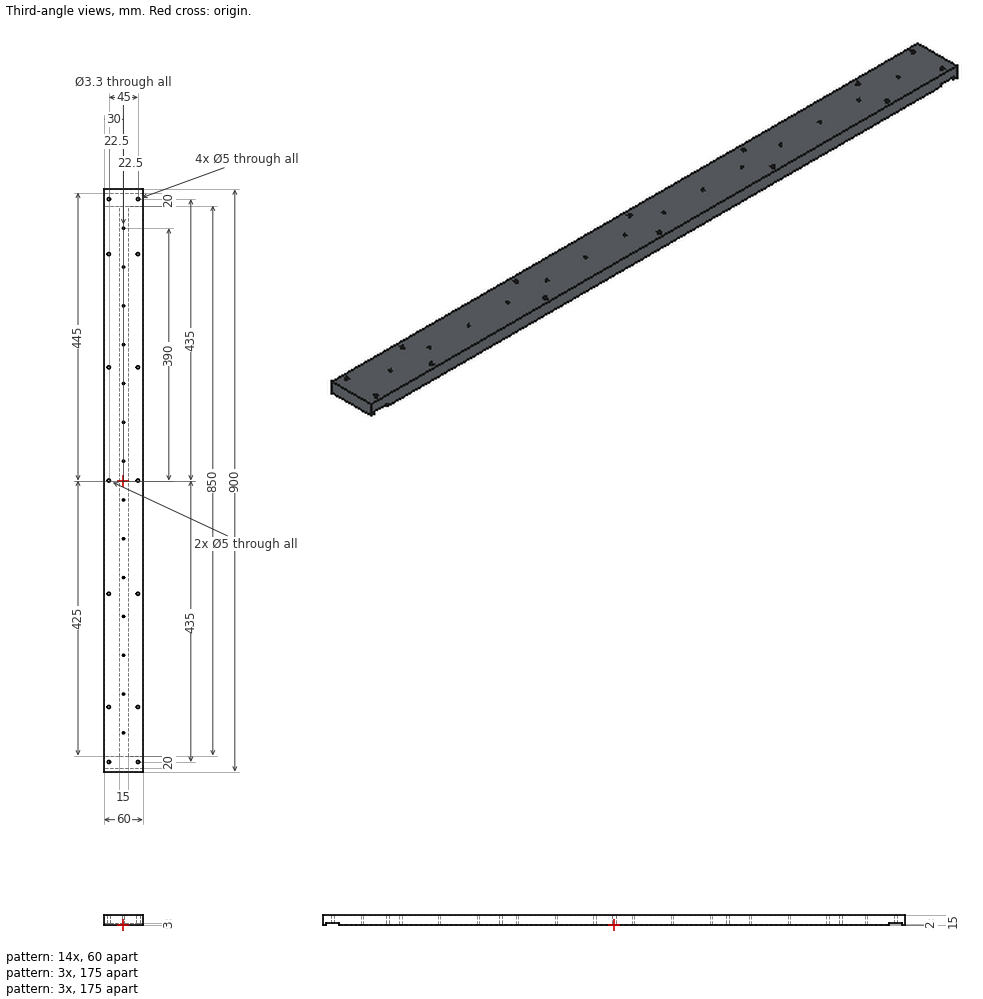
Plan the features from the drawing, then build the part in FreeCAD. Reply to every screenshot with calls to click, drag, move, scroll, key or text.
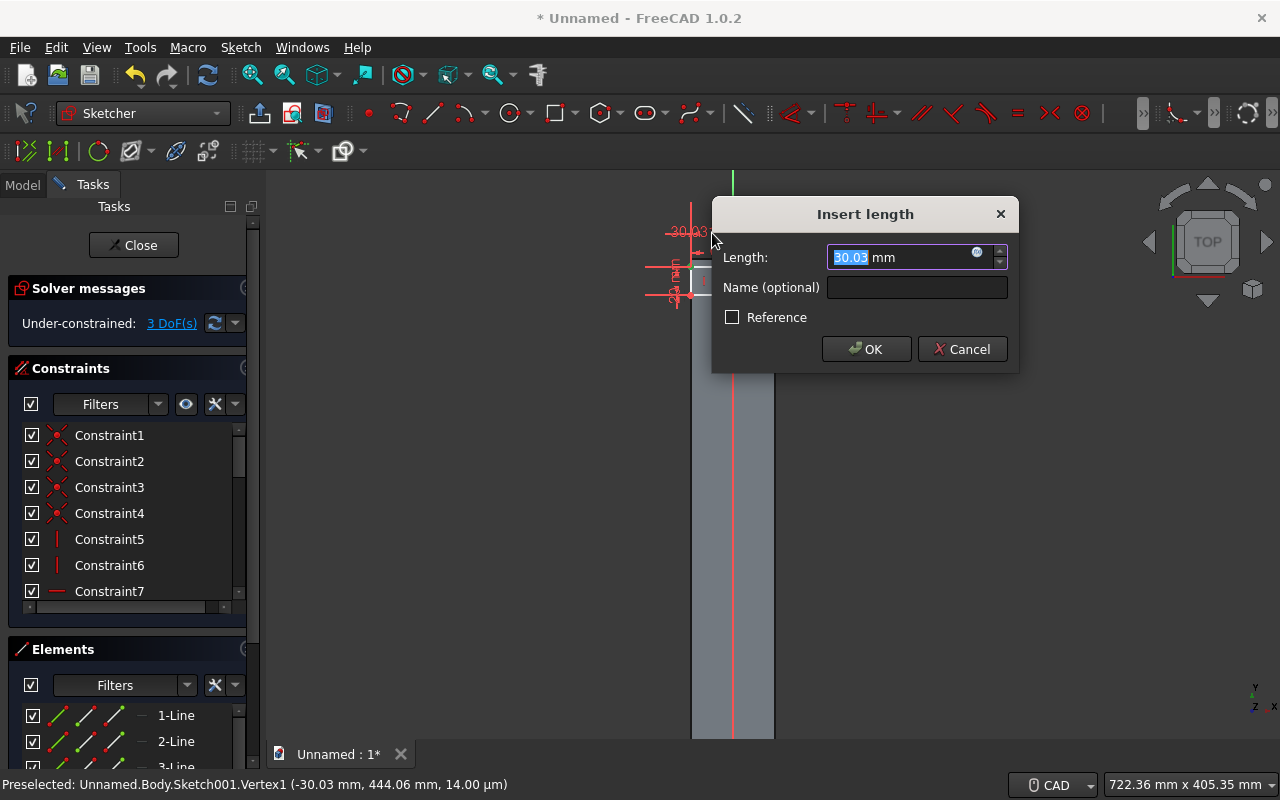
text(30)
key(Return)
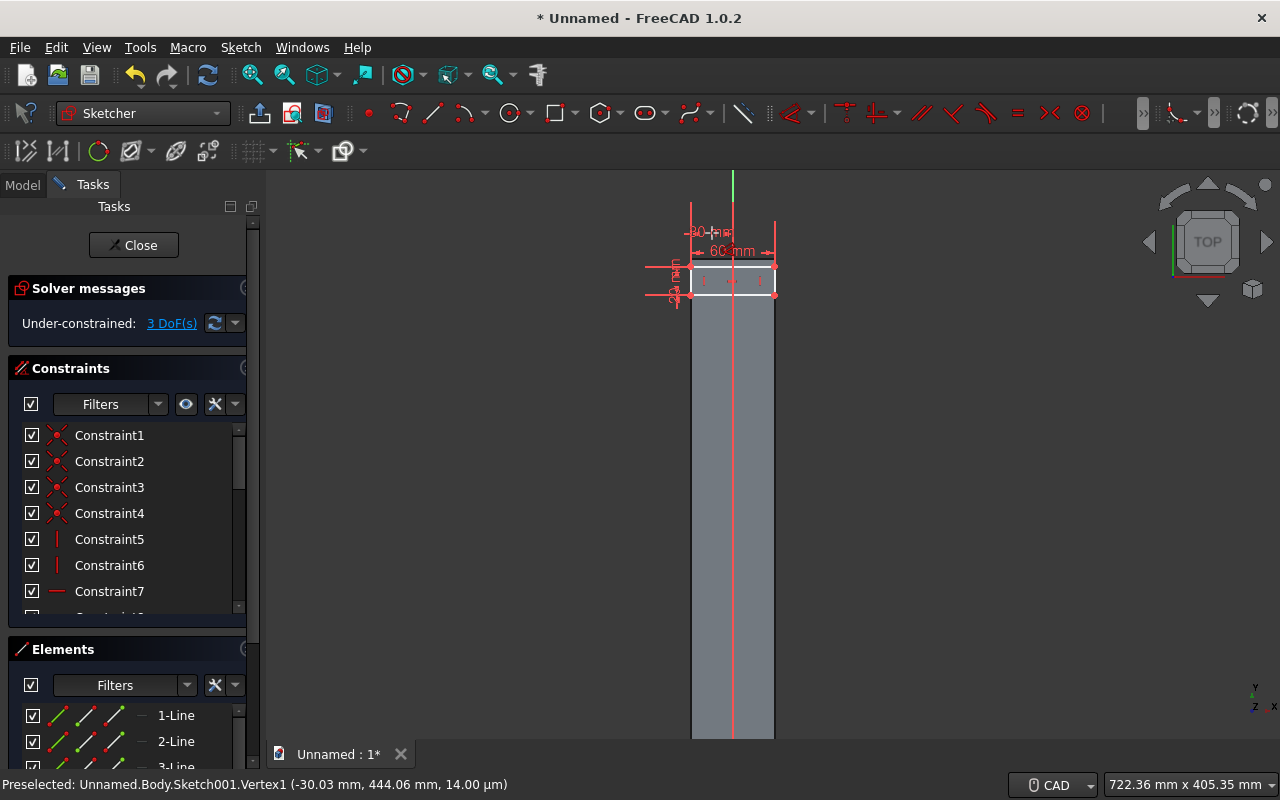
scroll(692, 267, down, 6)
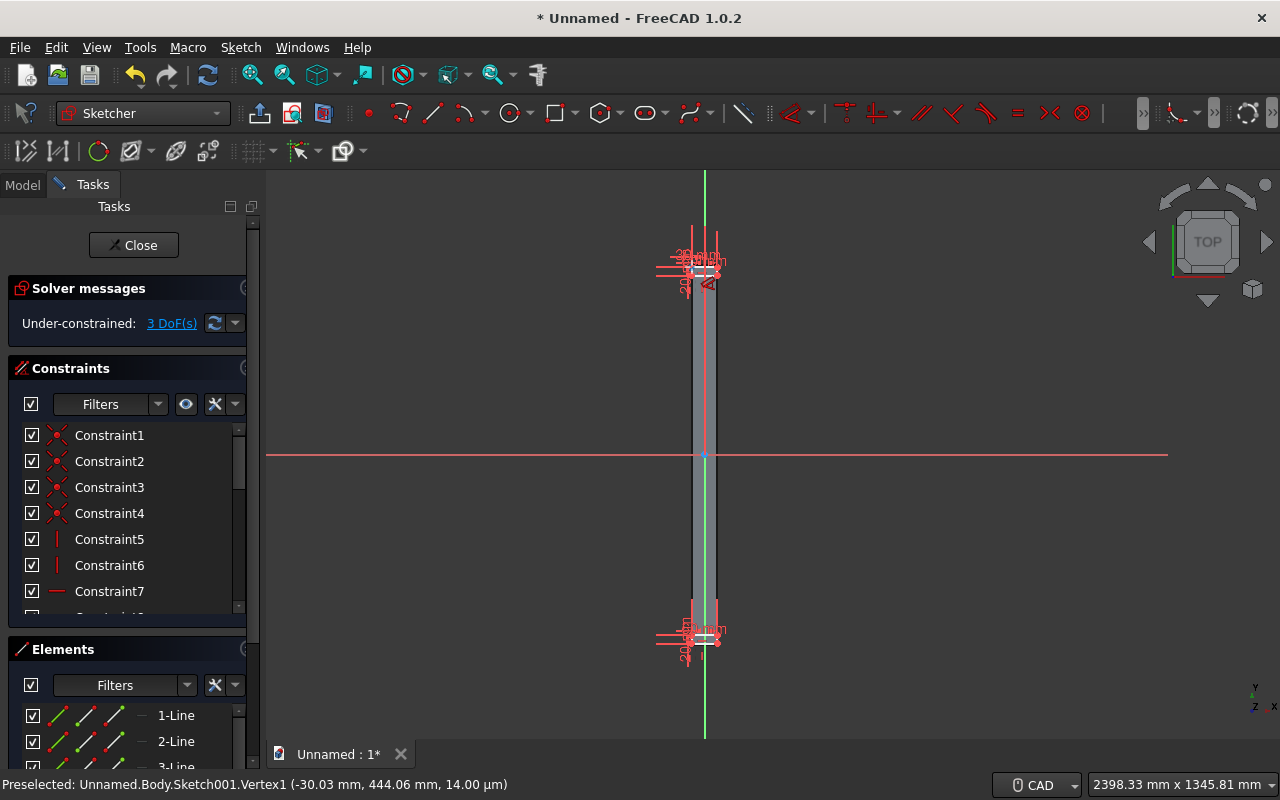
scroll(692, 635, up, 6)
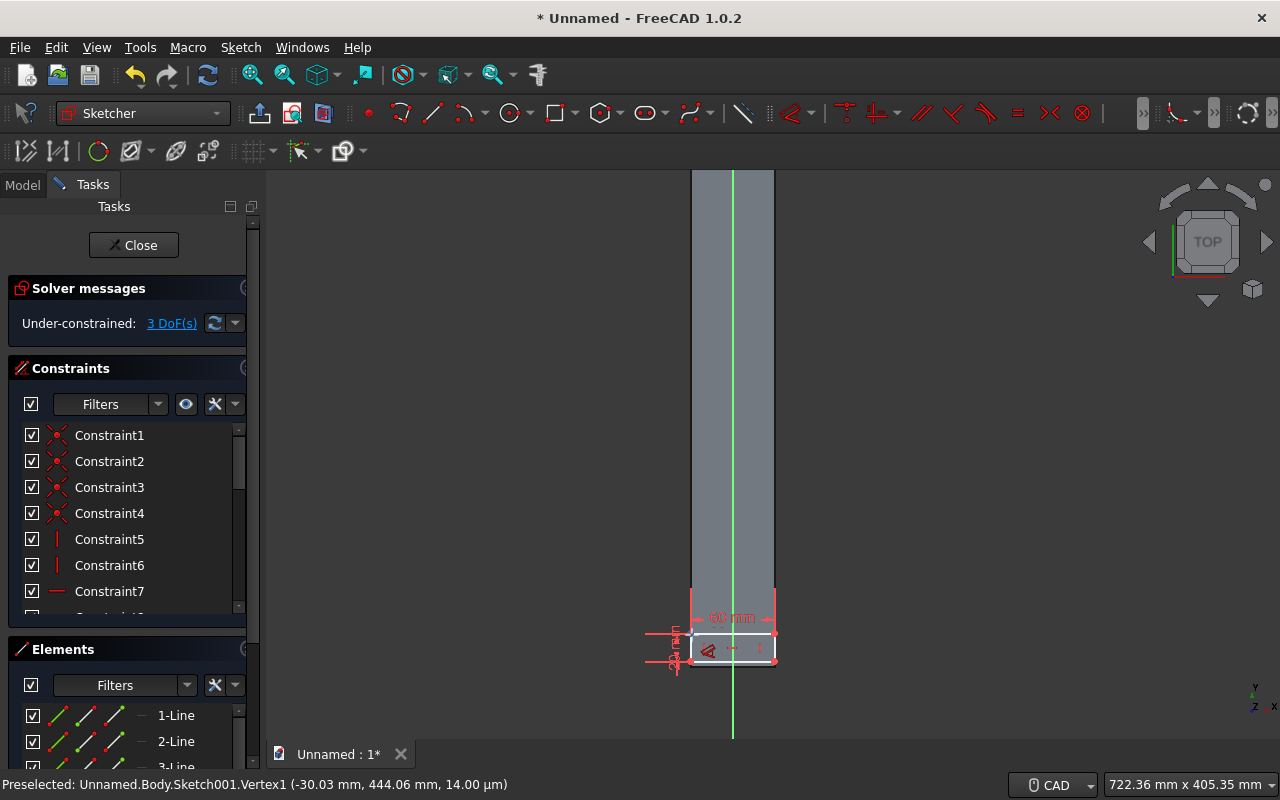
click(691, 634)
click(712, 692)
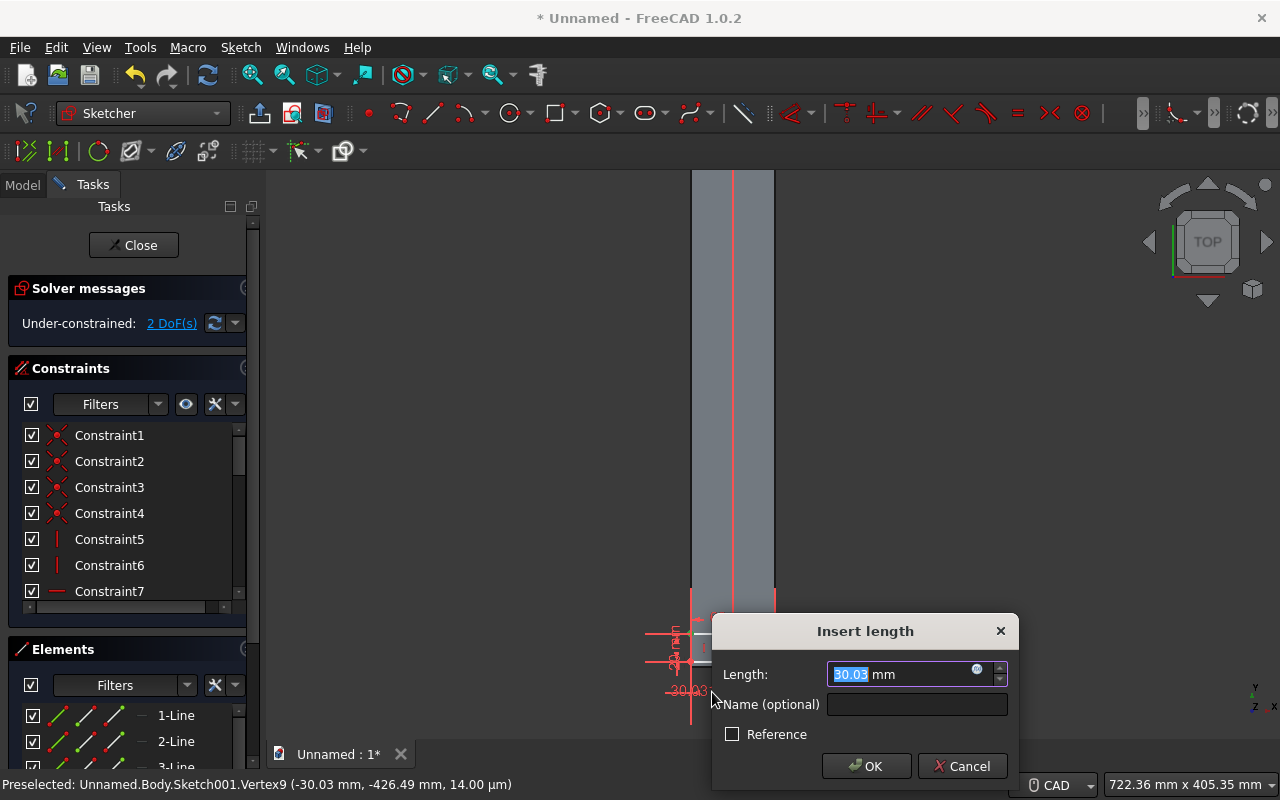
text(30)
key(Return)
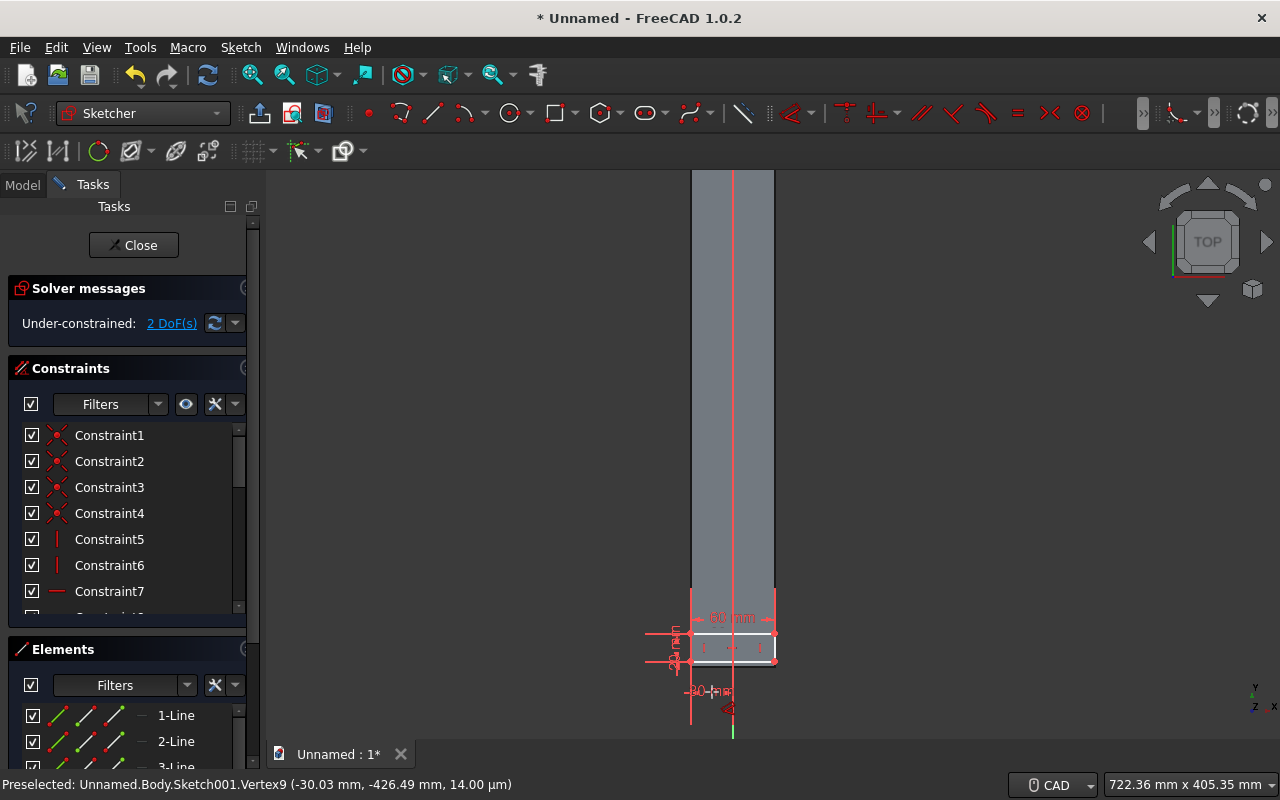
scroll(692, 635, down, 6)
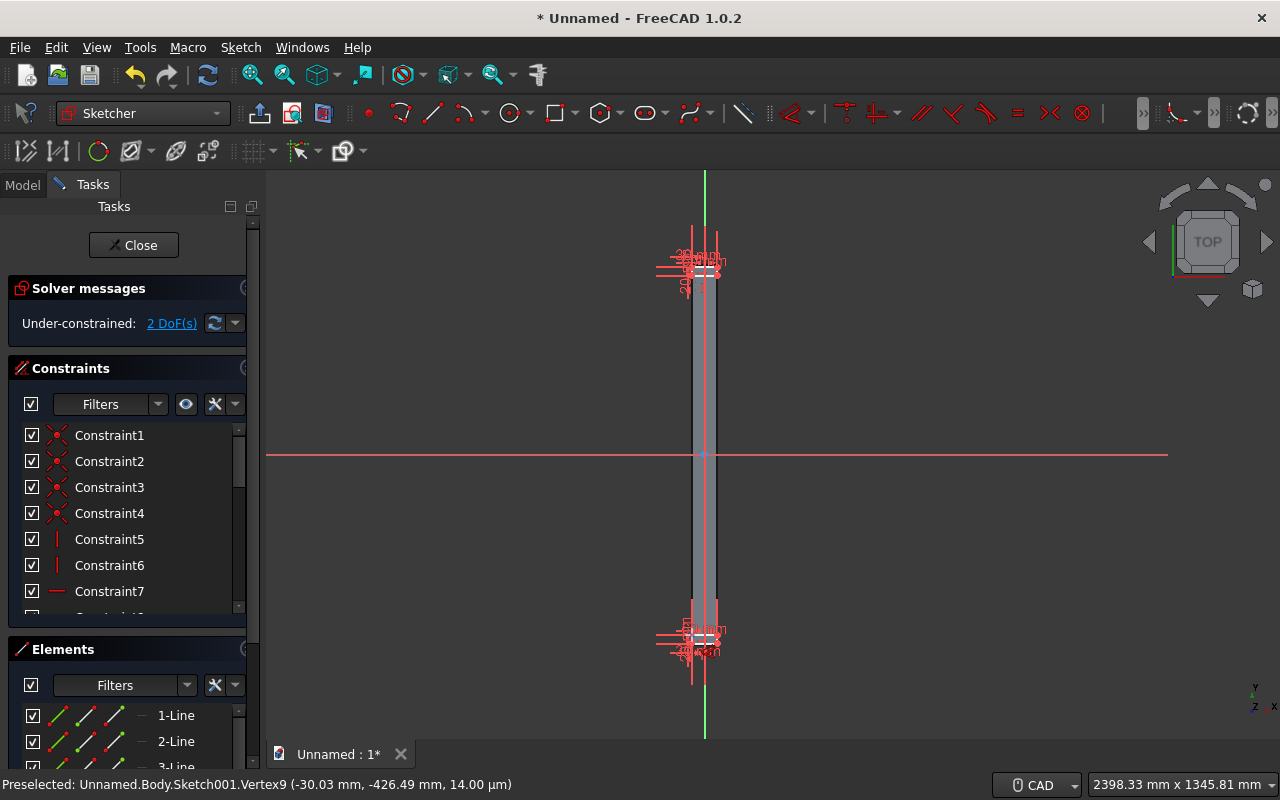
scroll(692, 267, up, 2)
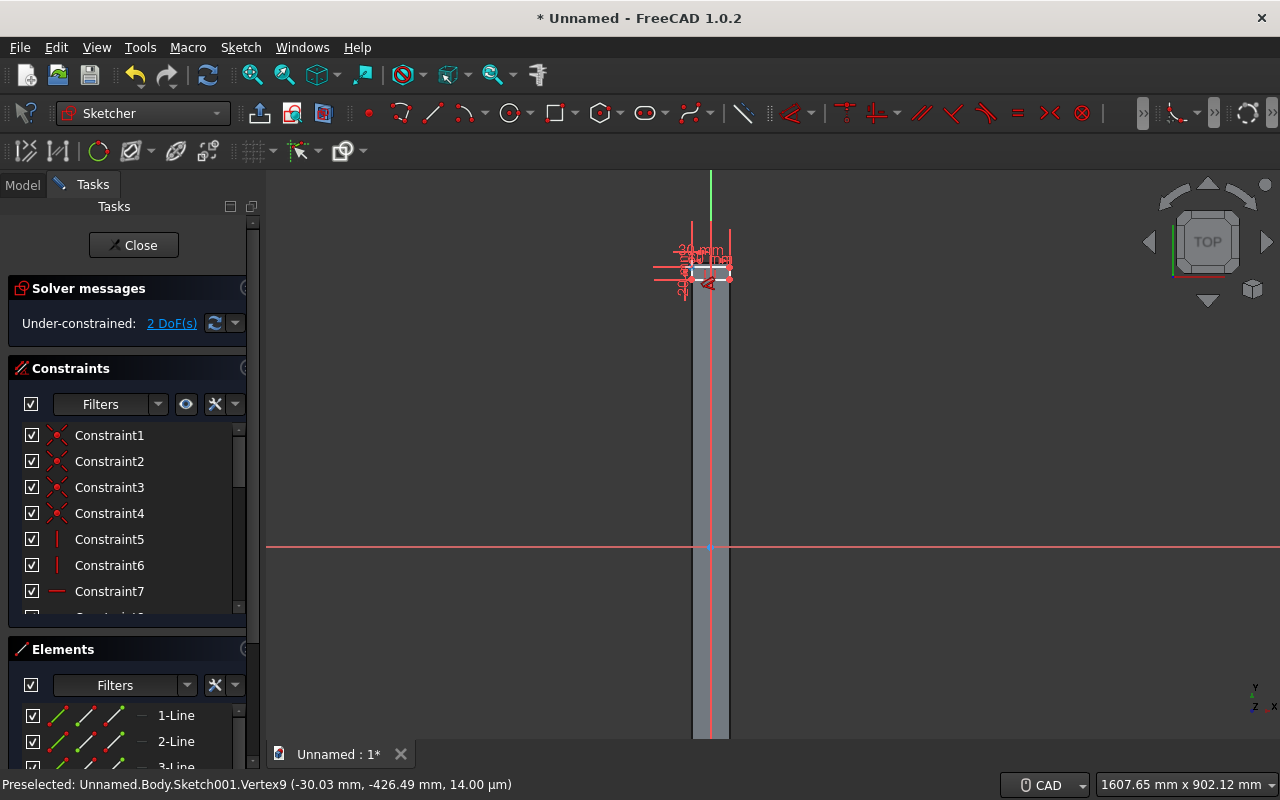
click(692, 267)
click(658, 407)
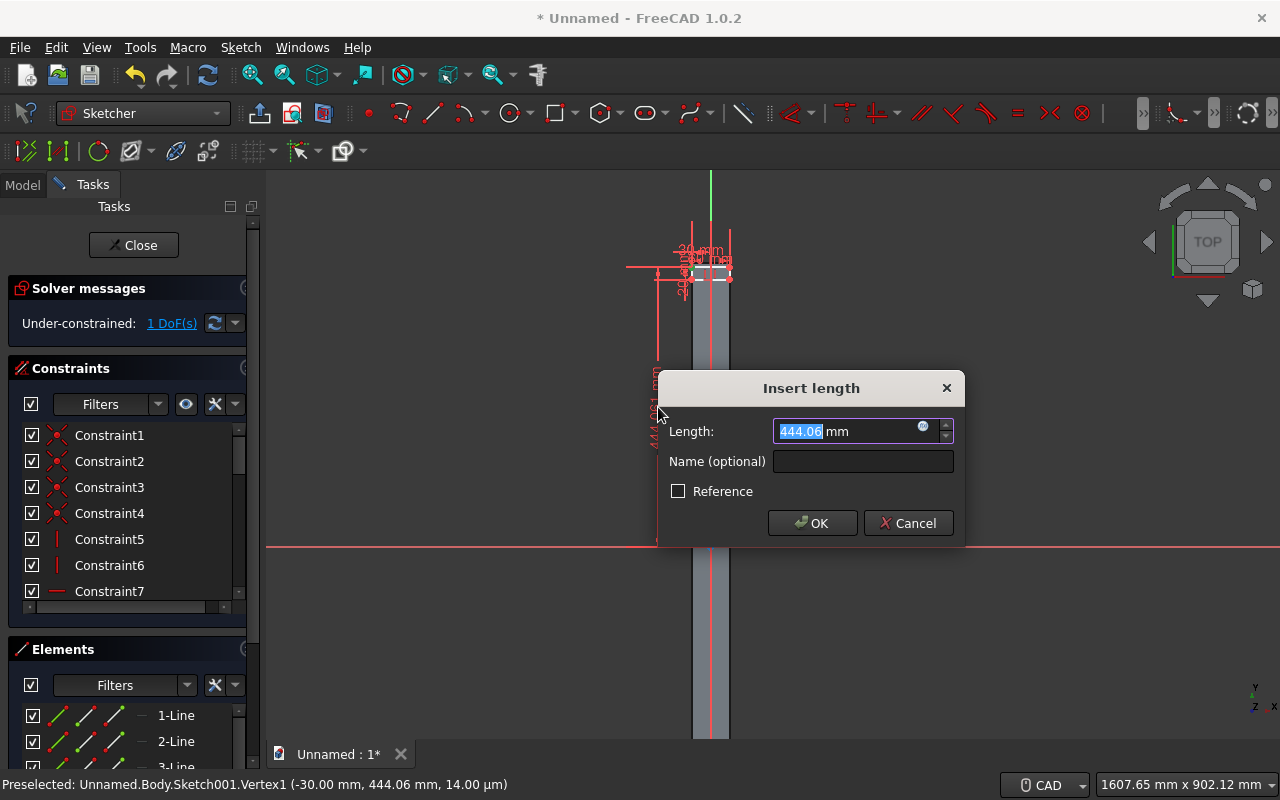
text(445)
key(Return)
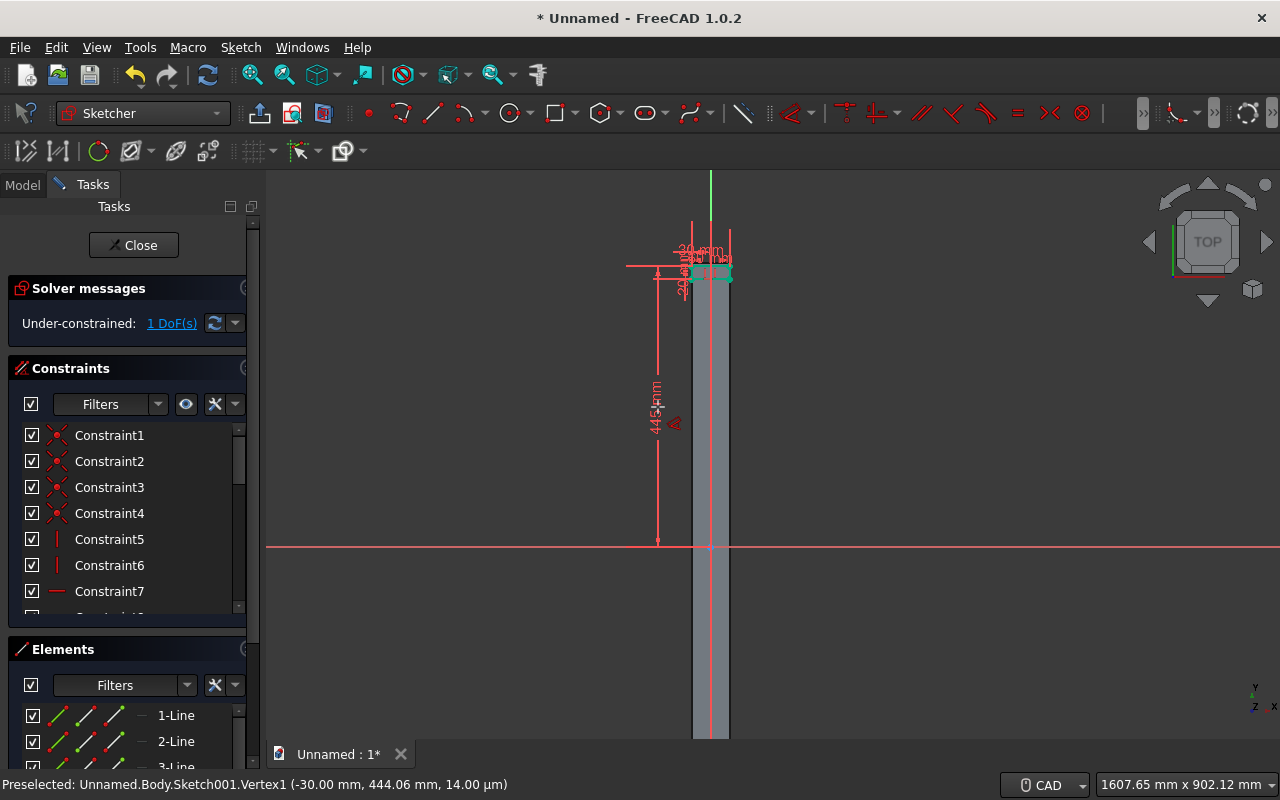
scroll(692, 266, down, 2)